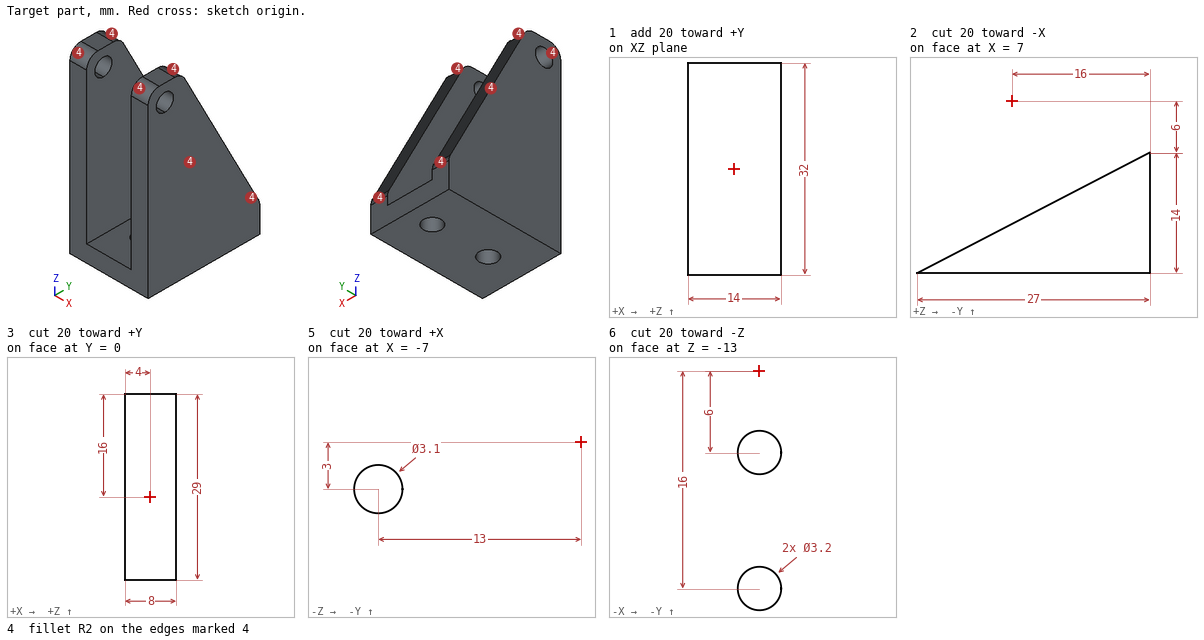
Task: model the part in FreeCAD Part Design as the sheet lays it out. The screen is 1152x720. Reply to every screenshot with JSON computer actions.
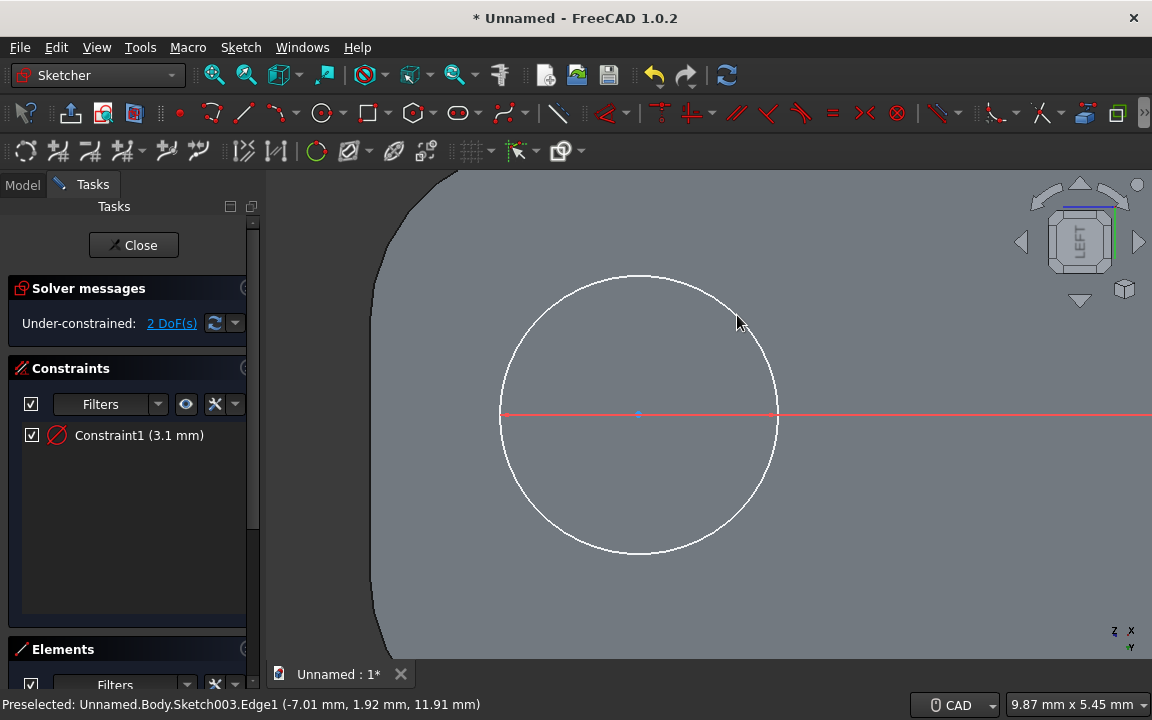
{"action": "left_click", "coordinate": [606, 114]}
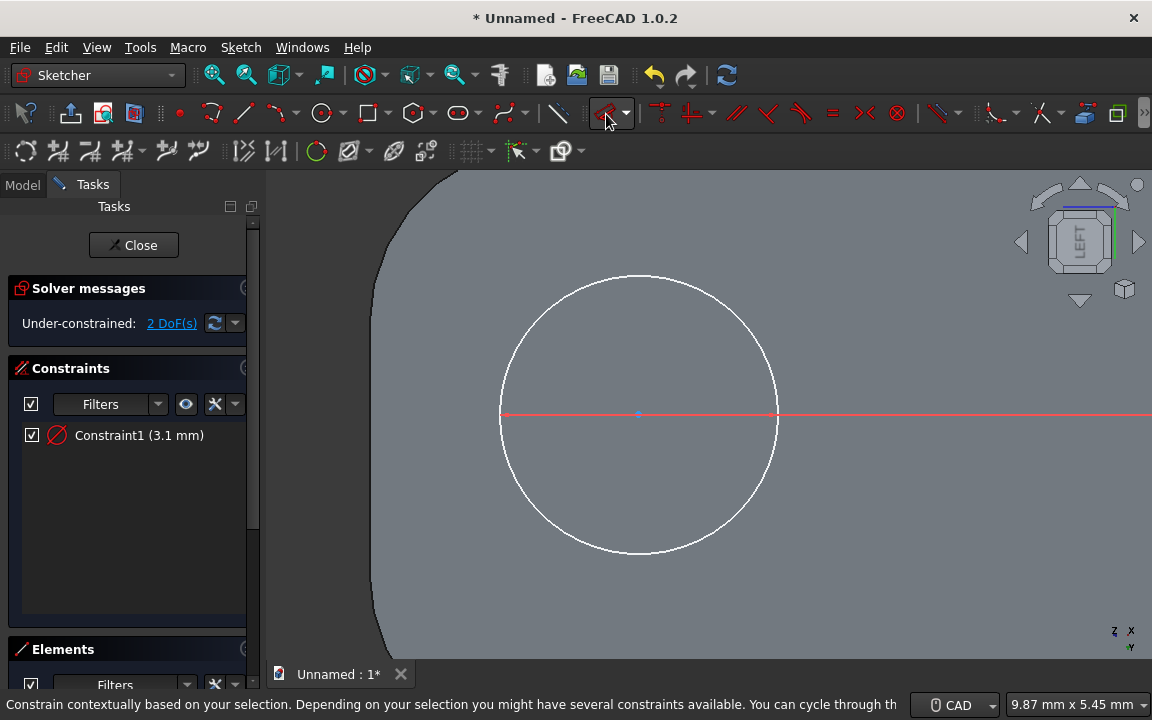
{"action": "left_click", "coordinate": [639, 415]}
{"action": "left_click", "coordinate": [605, 306]}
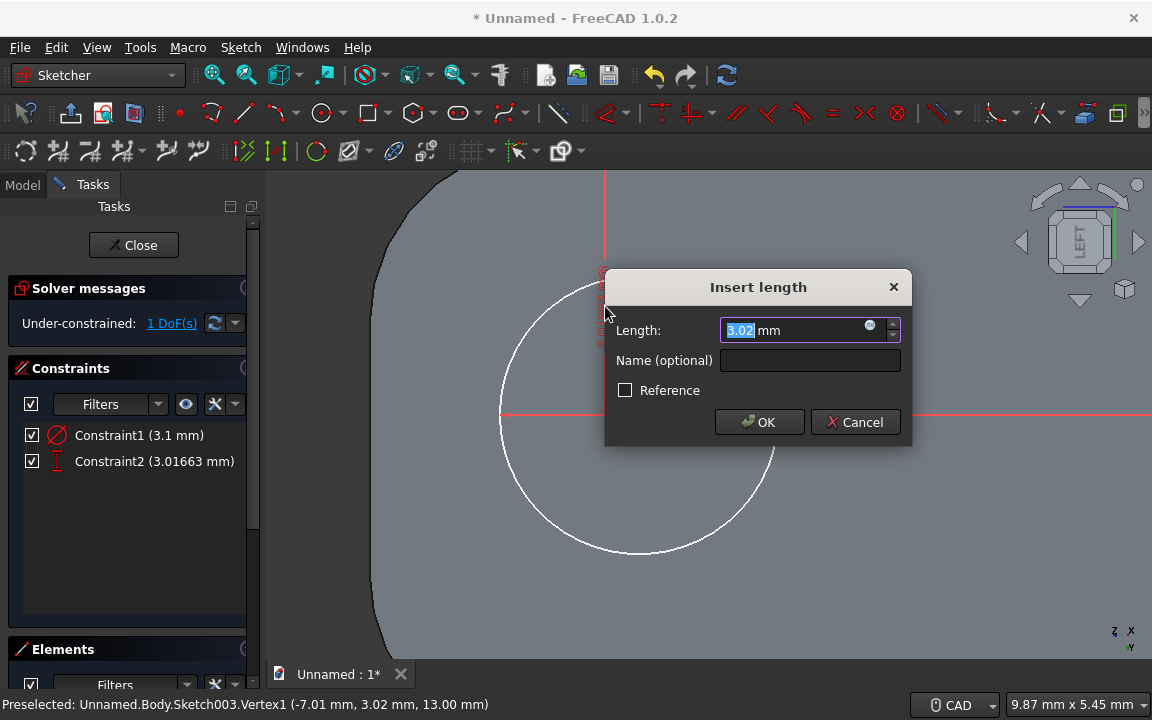
{"action": "type", "text": "3"}
{"action": "key", "text": "Return"}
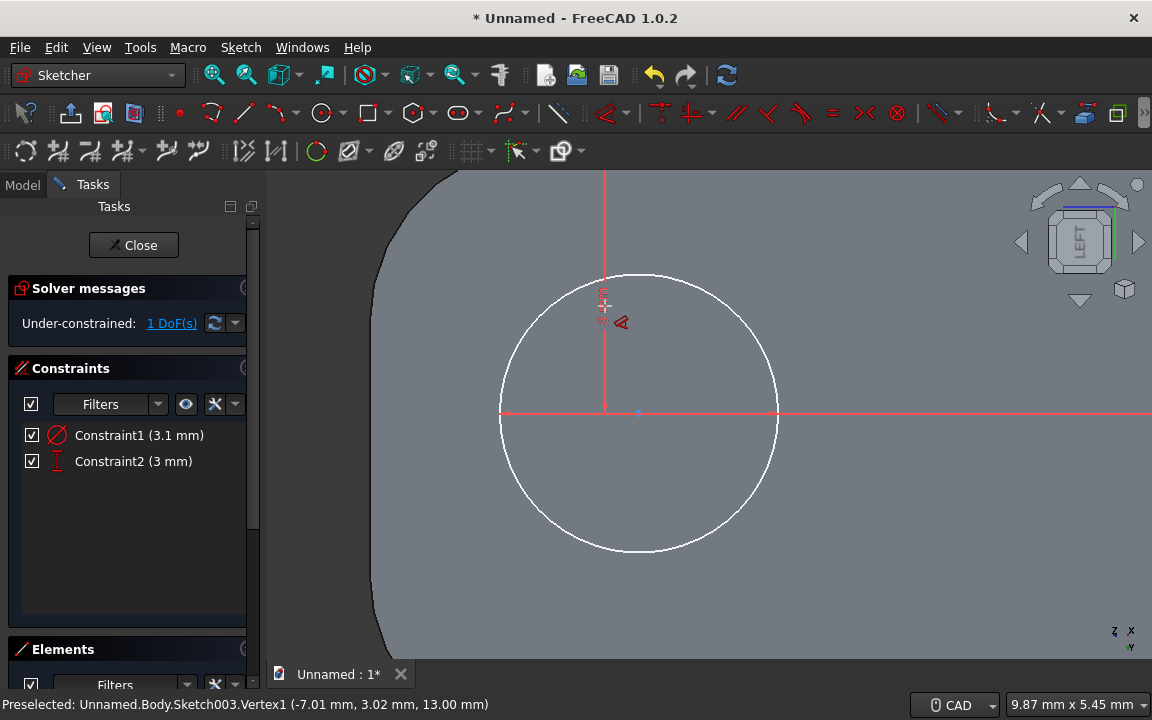
{"action": "left_click", "coordinate": [639, 414]}
{"action": "left_click", "coordinate": [813, 448]}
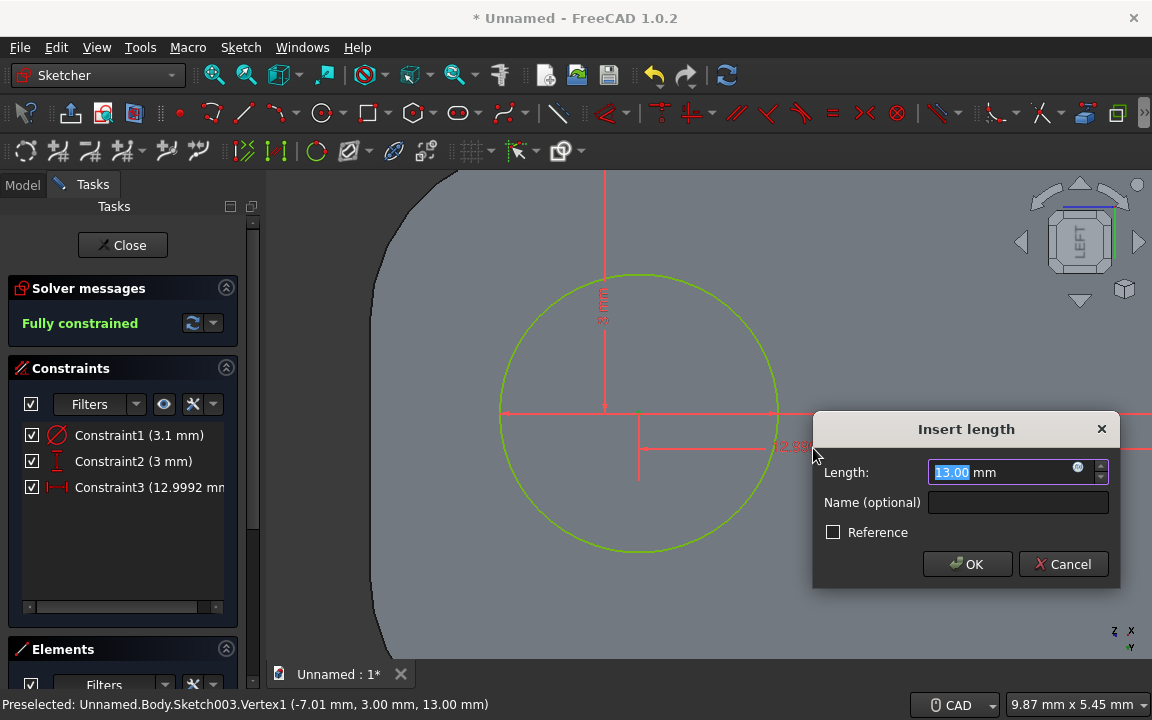
{"action": "type", "text": "13"}
{"action": "key", "text": "Return"}
{"action": "key", "text": "Escape"}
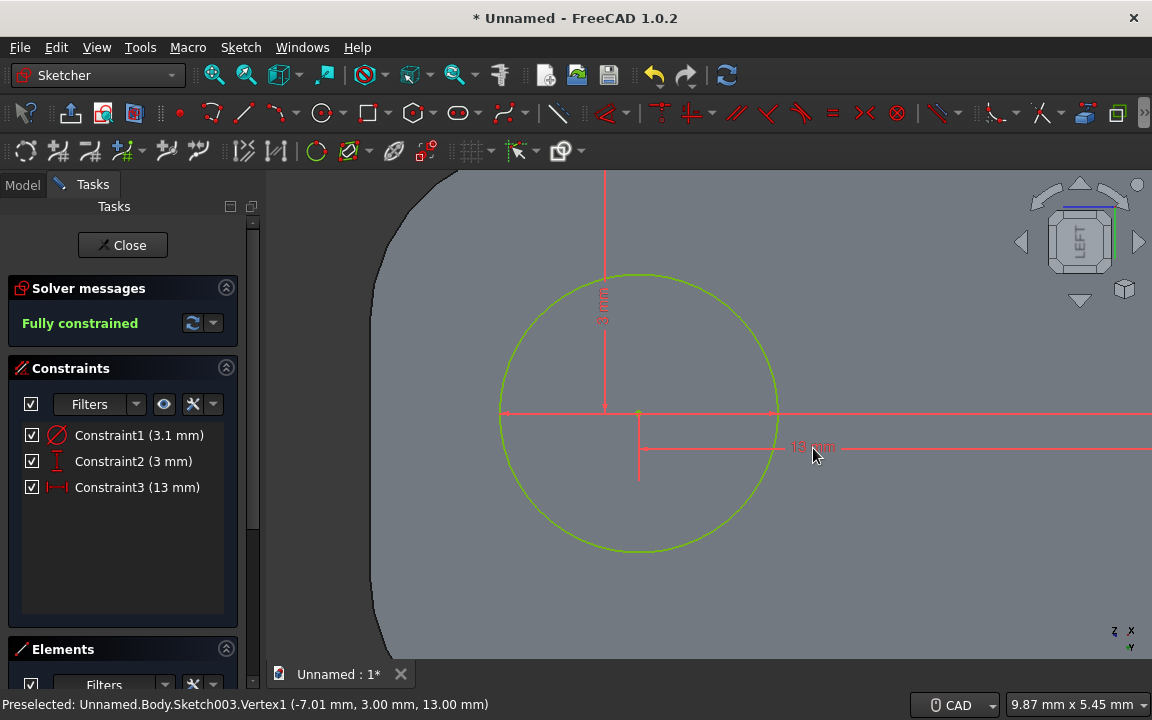
{"action": "left_click", "coordinate": [123, 245]}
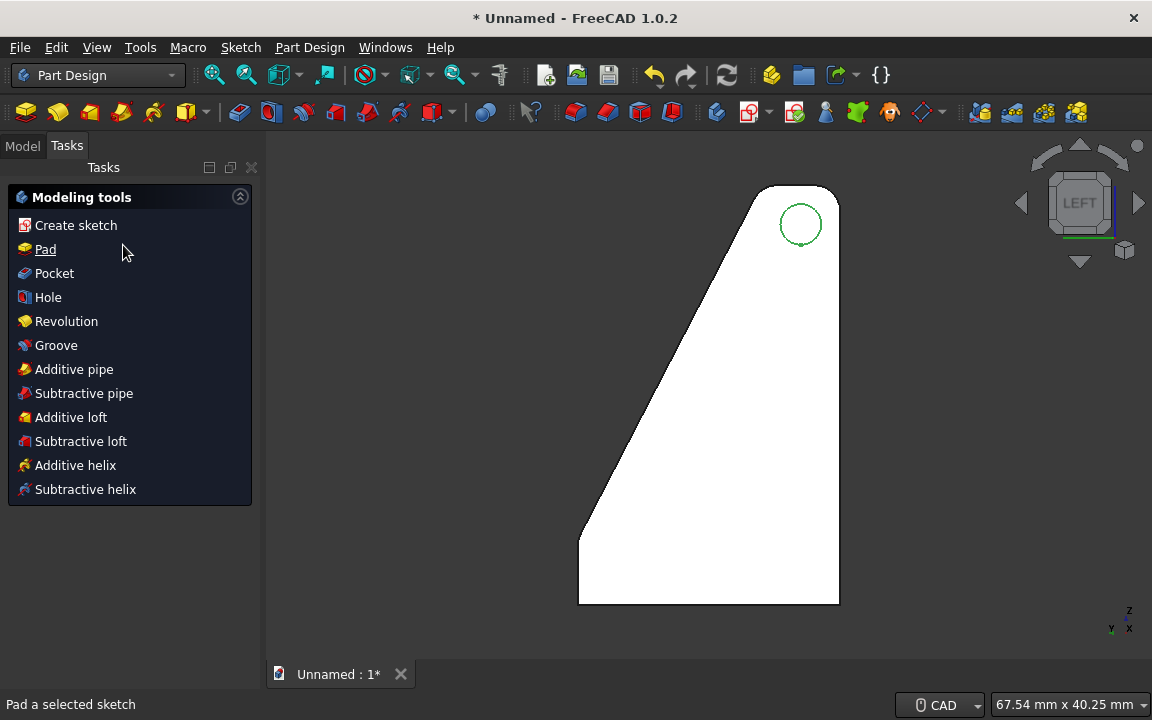
{"action": "left_click", "coordinate": [240, 112]}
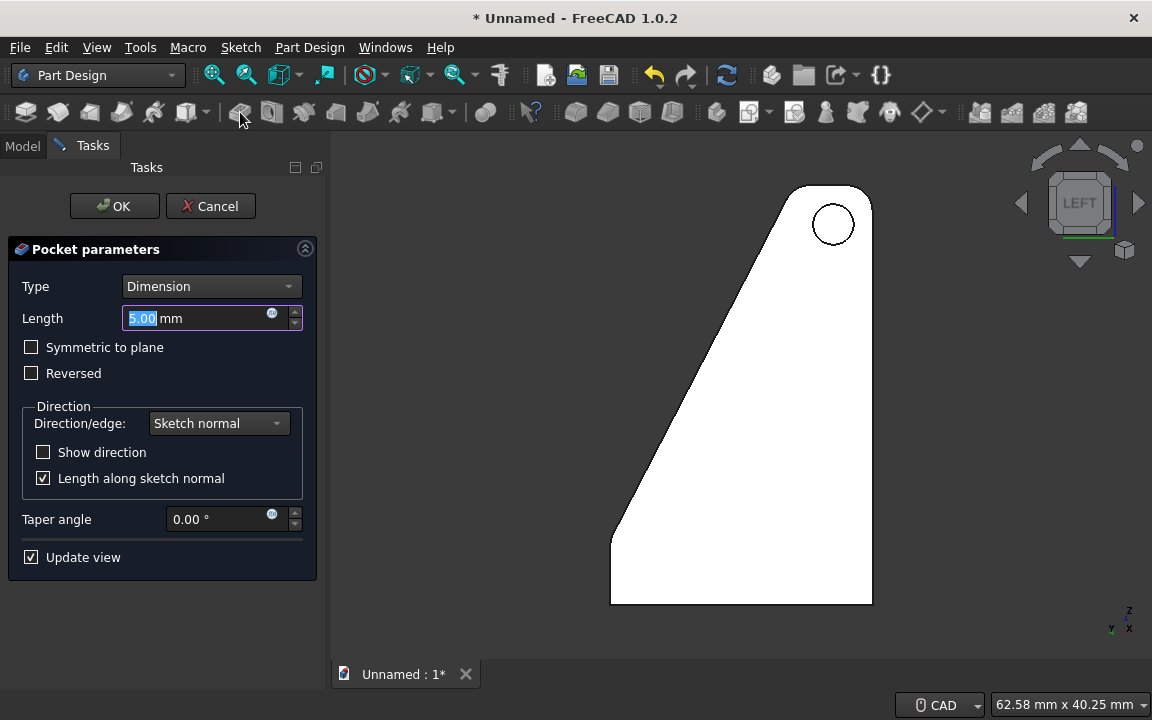
{"action": "type", "text": "20"}
{"action": "key", "text": "Tab"}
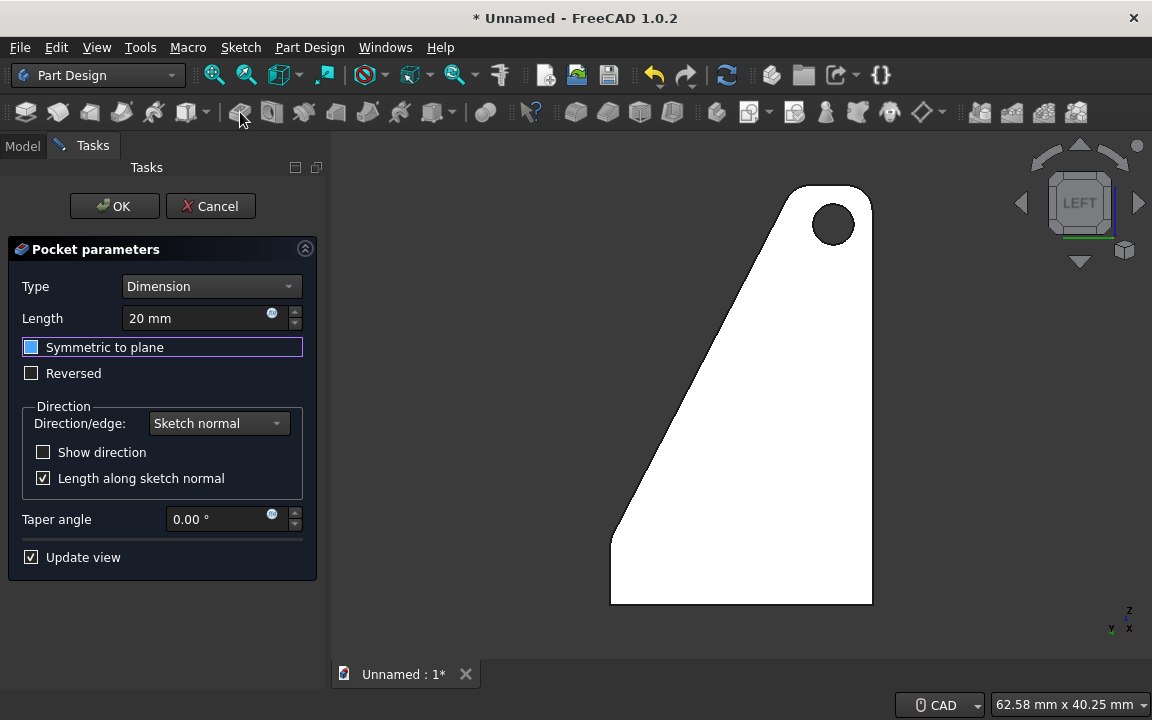
{"action": "left_click", "coordinate": [115, 206]}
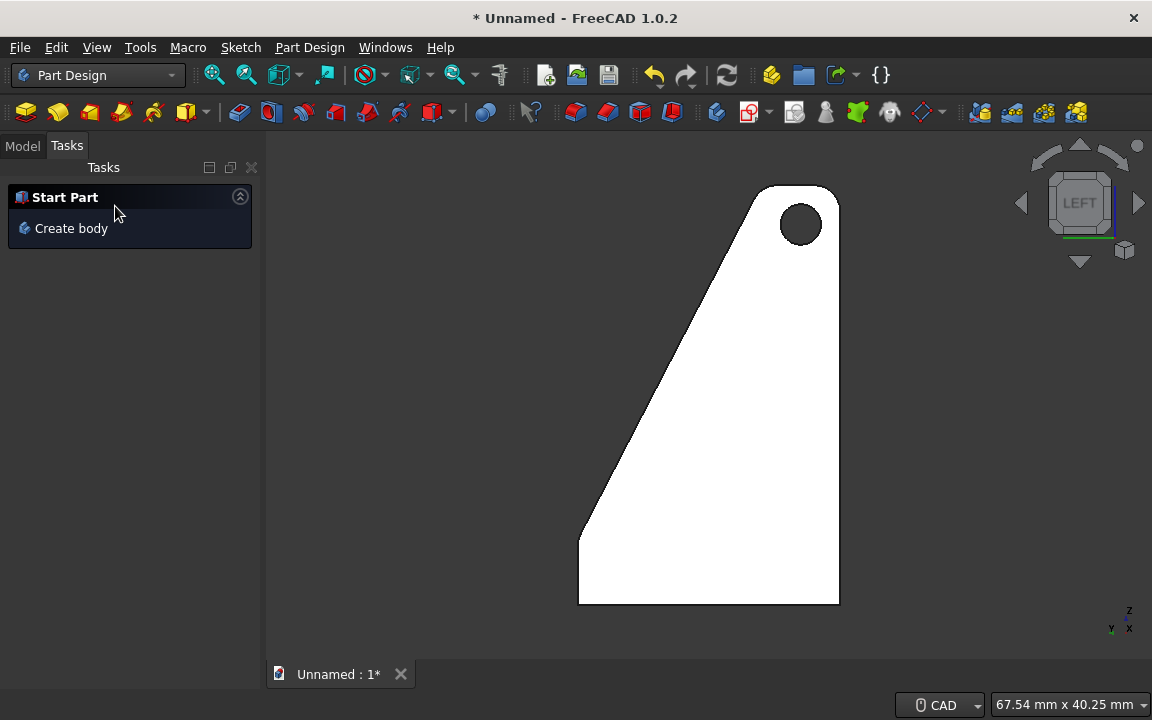
{"action": "key", "text": "0"}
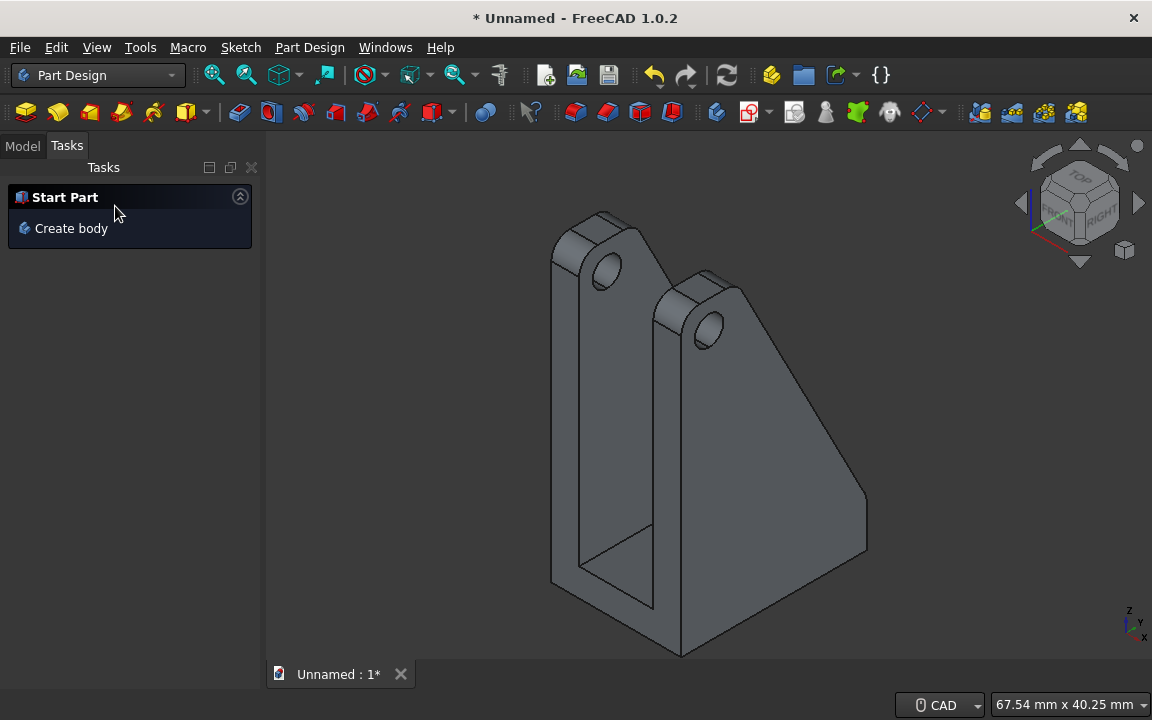
{"action": "key", "text": "2"}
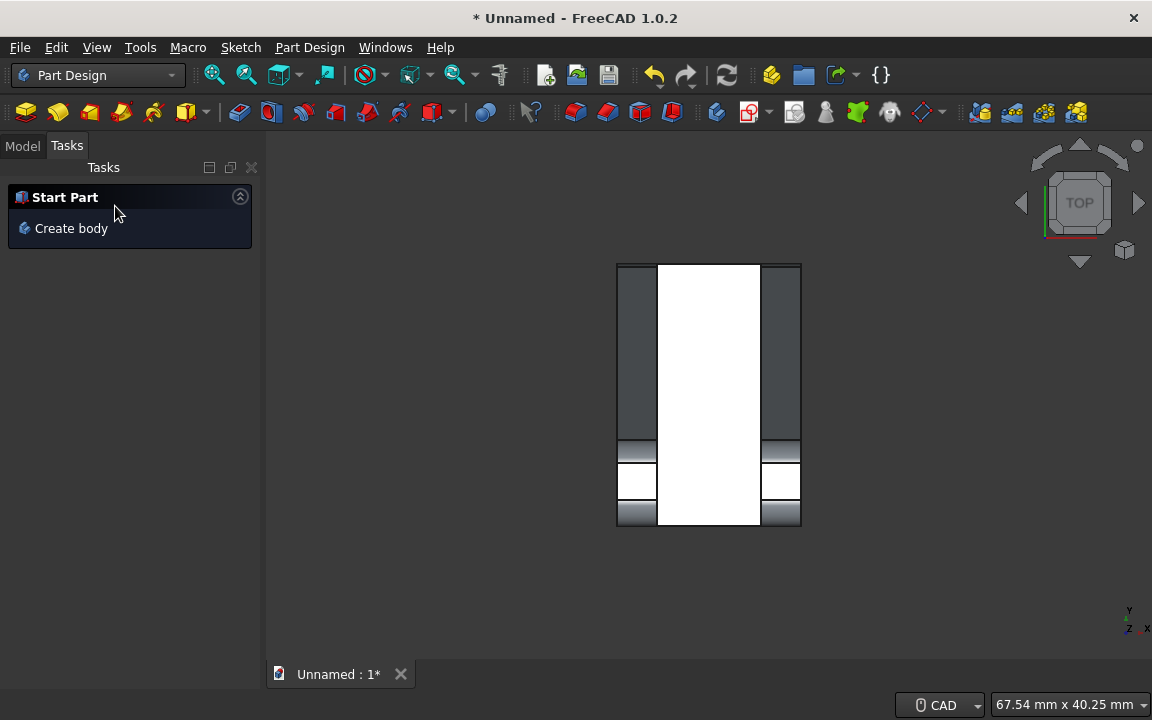
{"action": "left_click", "coordinate": [709, 319]}